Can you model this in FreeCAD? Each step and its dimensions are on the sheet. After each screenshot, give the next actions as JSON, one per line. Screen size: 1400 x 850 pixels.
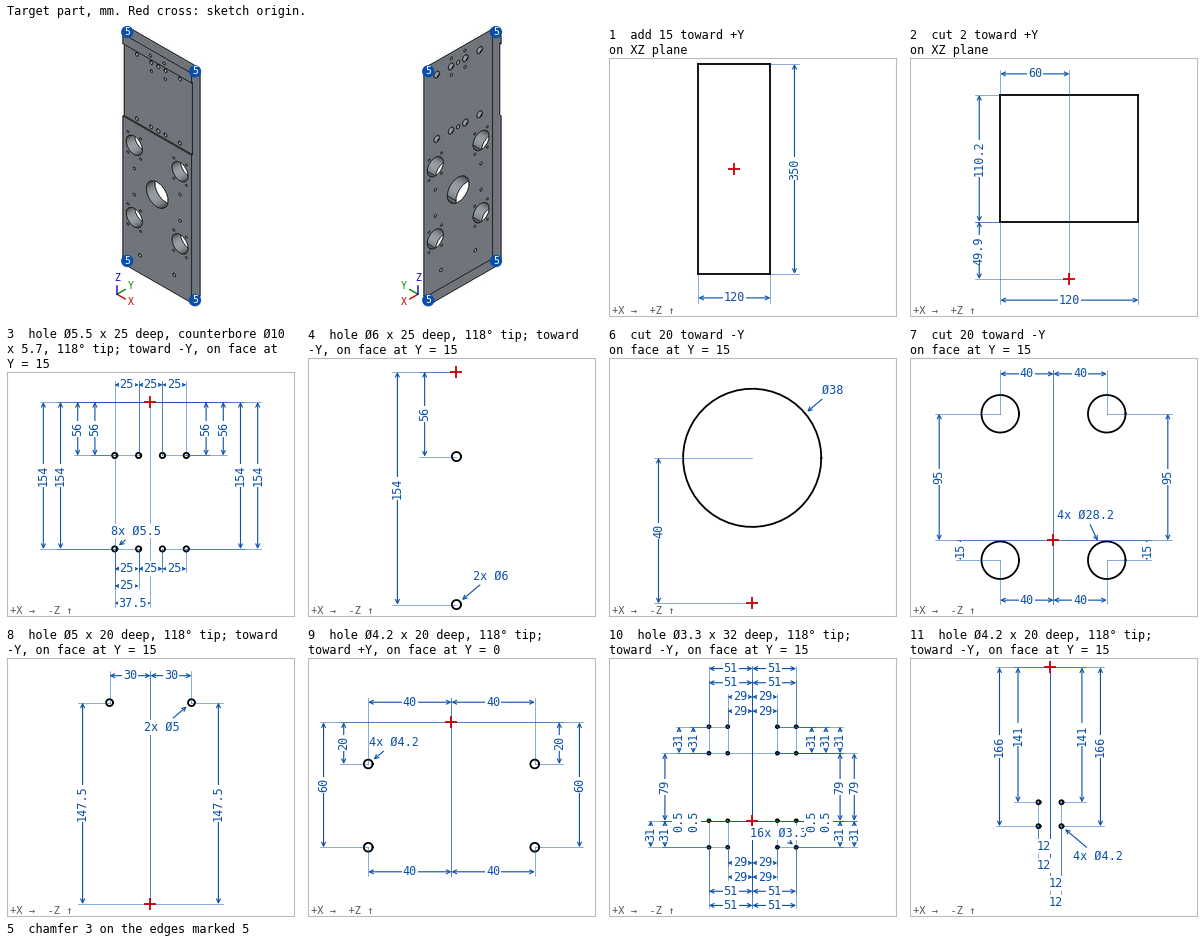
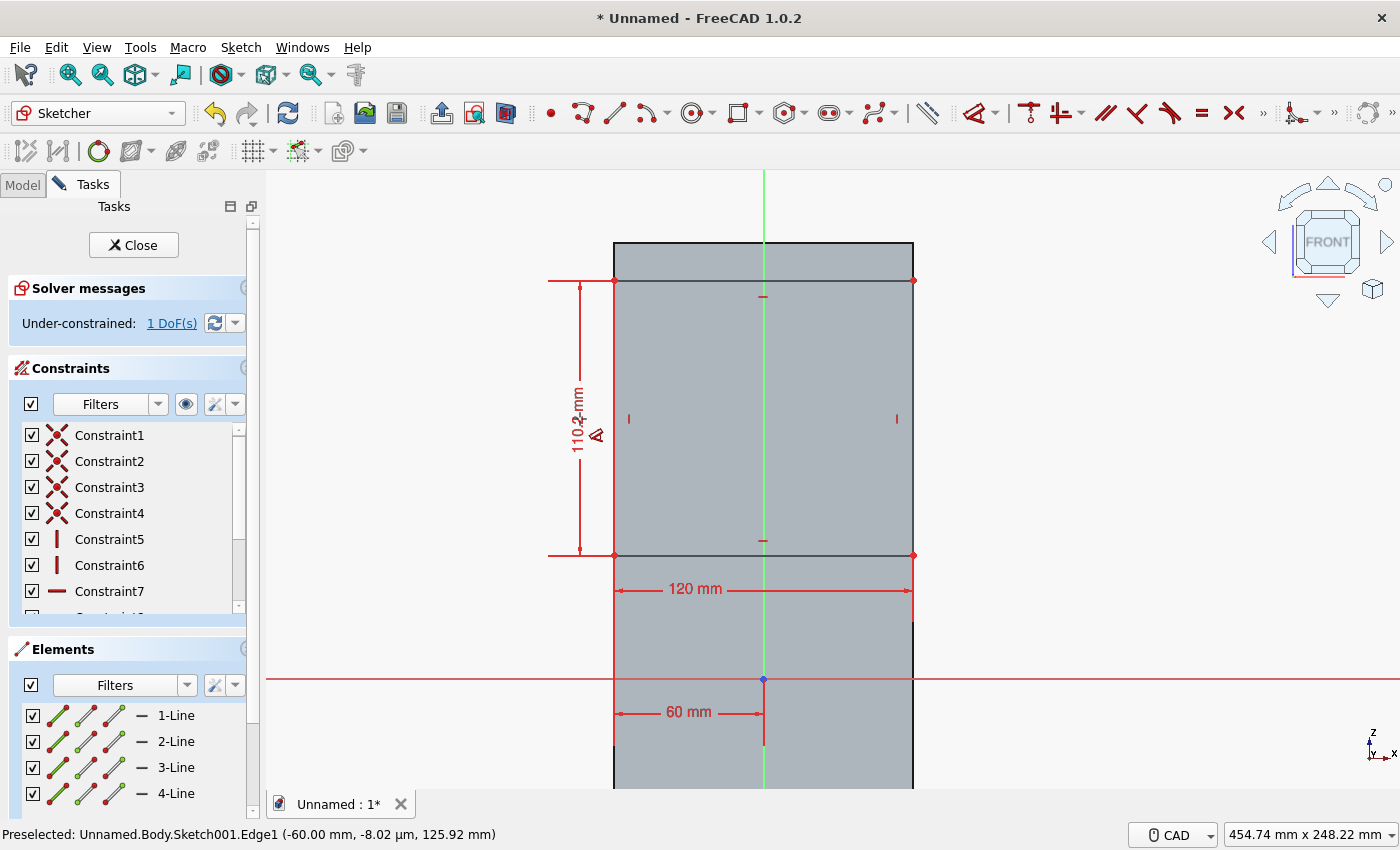
{"action": "left_click", "coordinate": [614, 556]}
{"action": "left_click", "coordinate": [580, 617]}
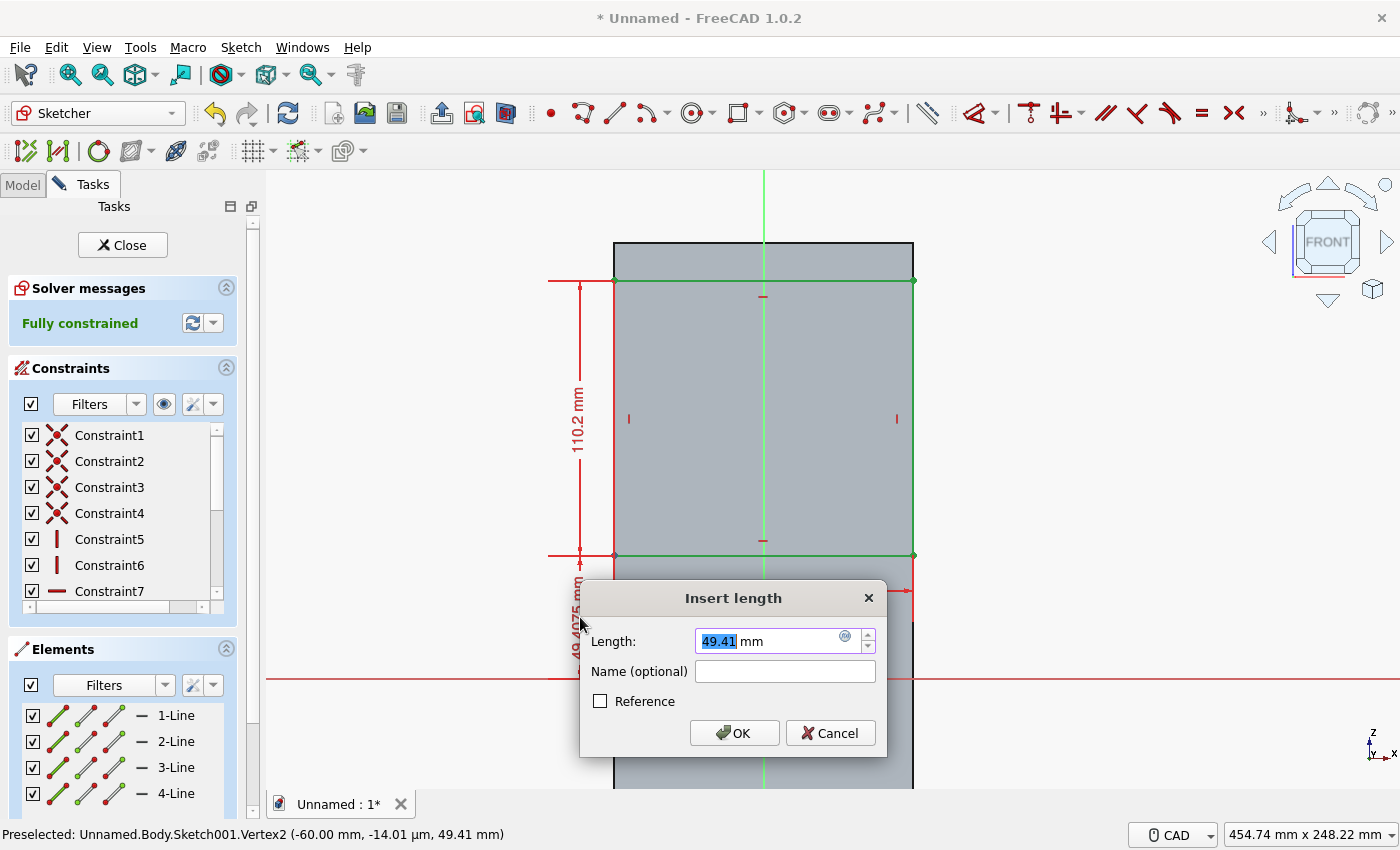
{"action": "type", "text": "49.9"}
{"action": "key", "text": "Return"}
{"action": "key", "text": "Escape"}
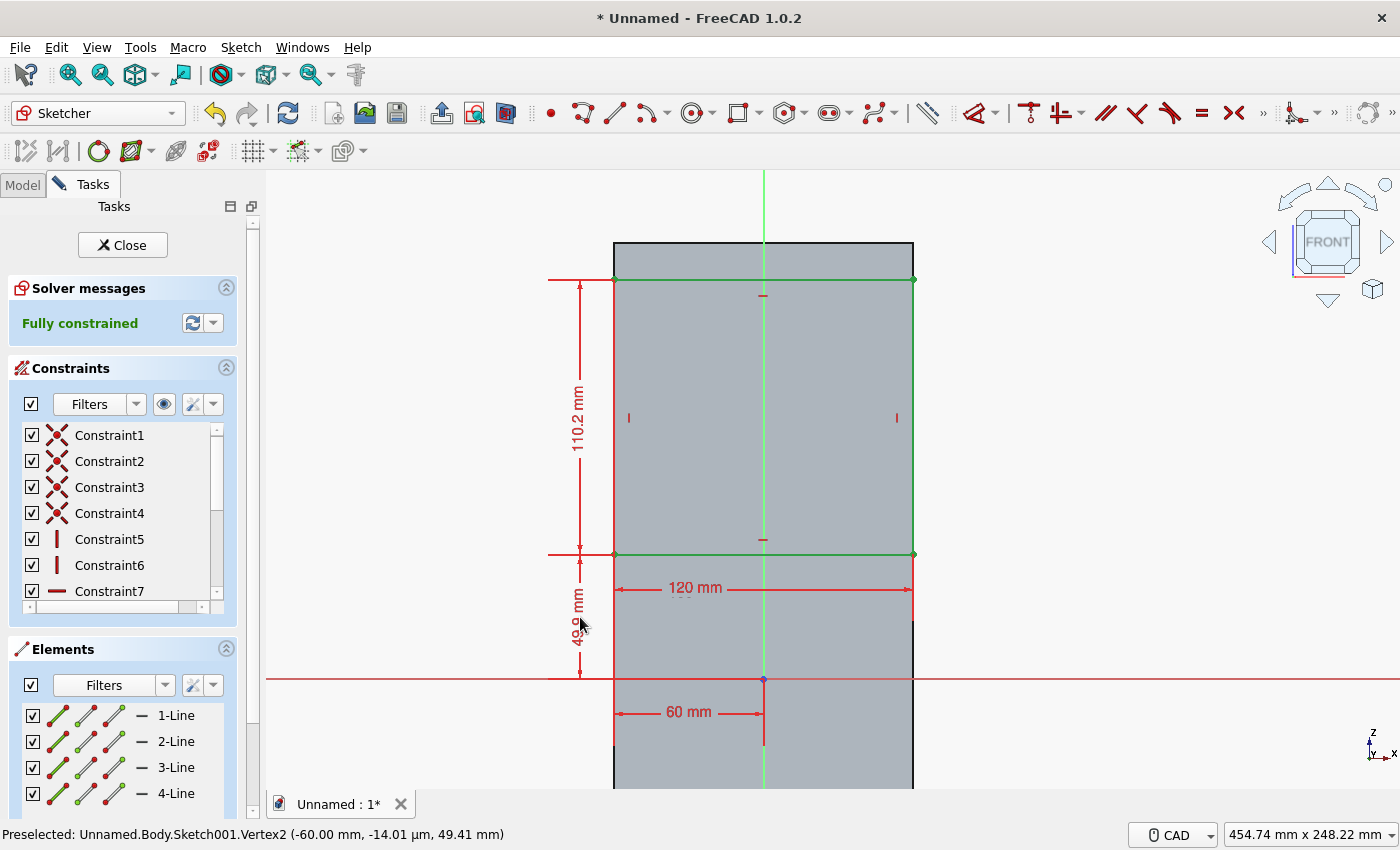
{"action": "left_click", "coordinate": [123, 245]}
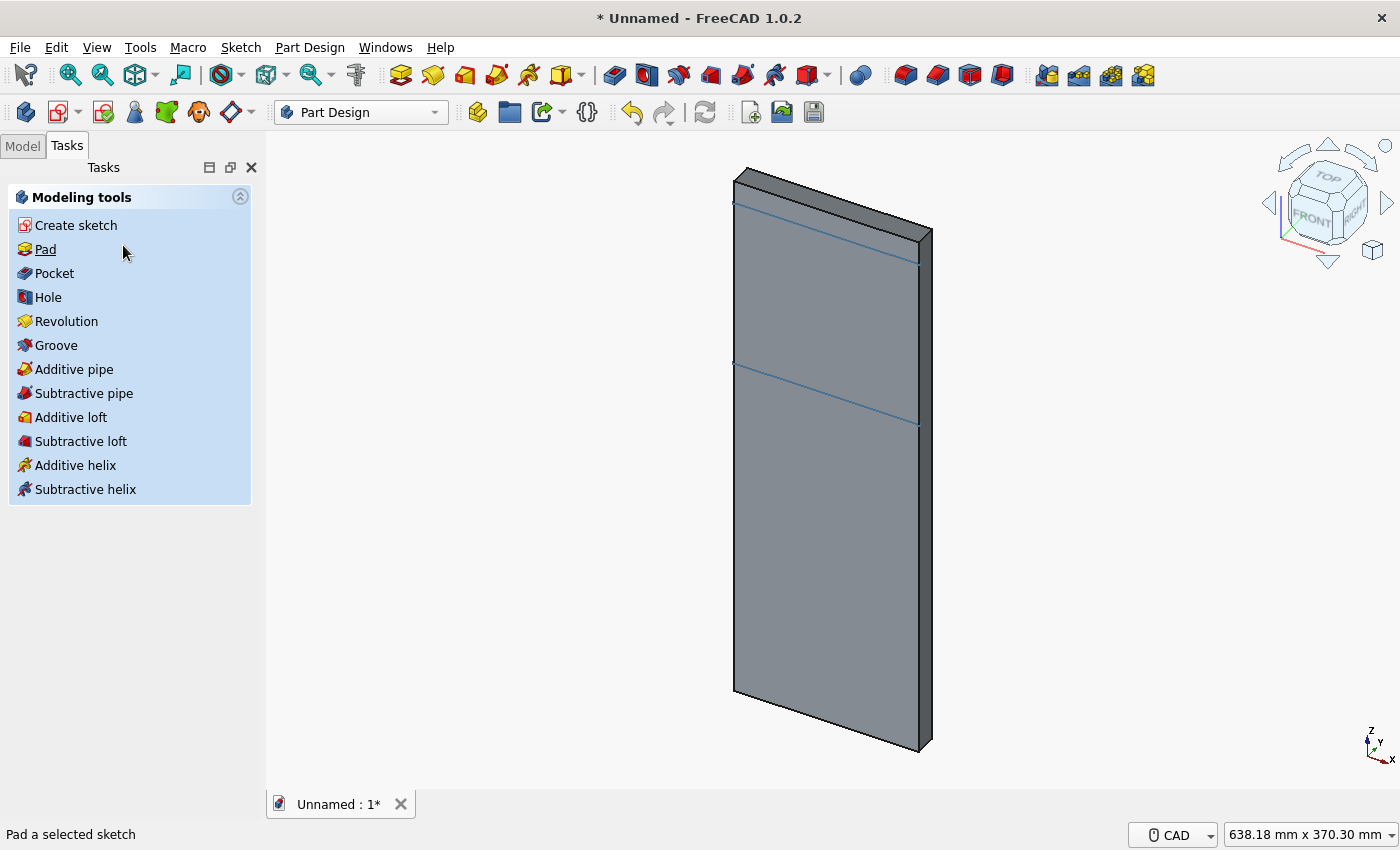
{"action": "left_click", "coordinate": [616, 76]}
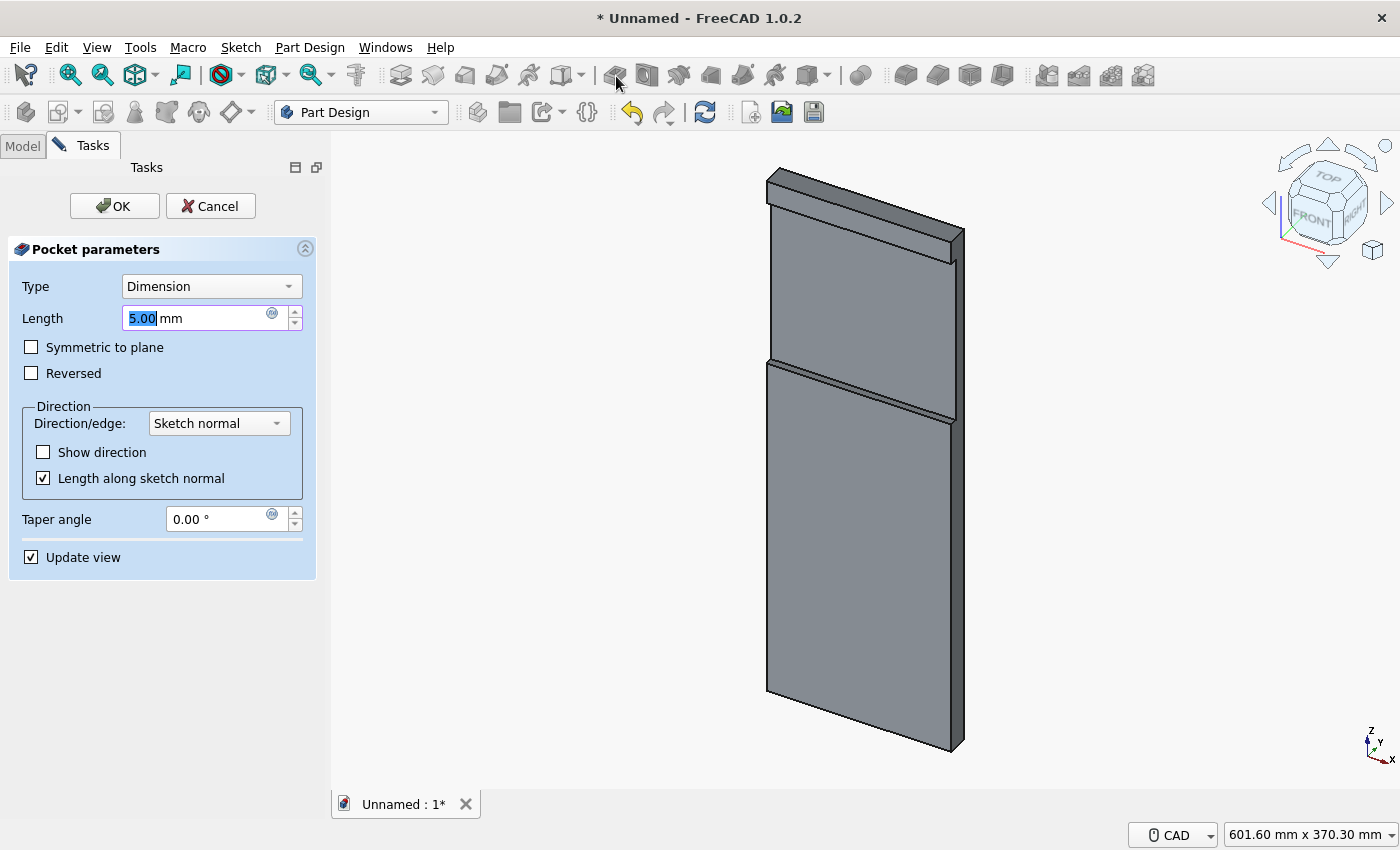
{"action": "type", "text": "2"}
{"action": "key", "text": "Tab"}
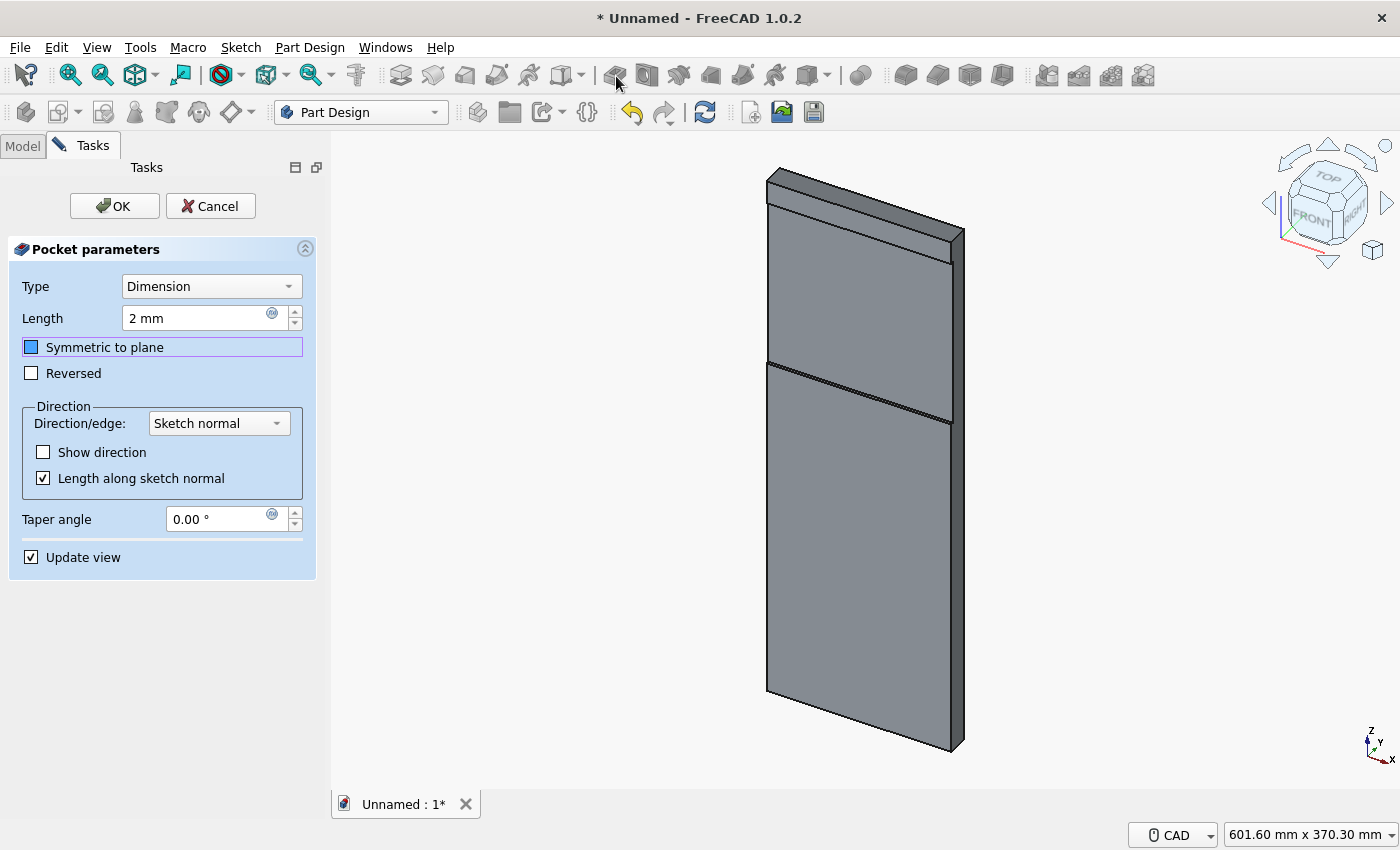
{"action": "left_click", "coordinate": [115, 206]}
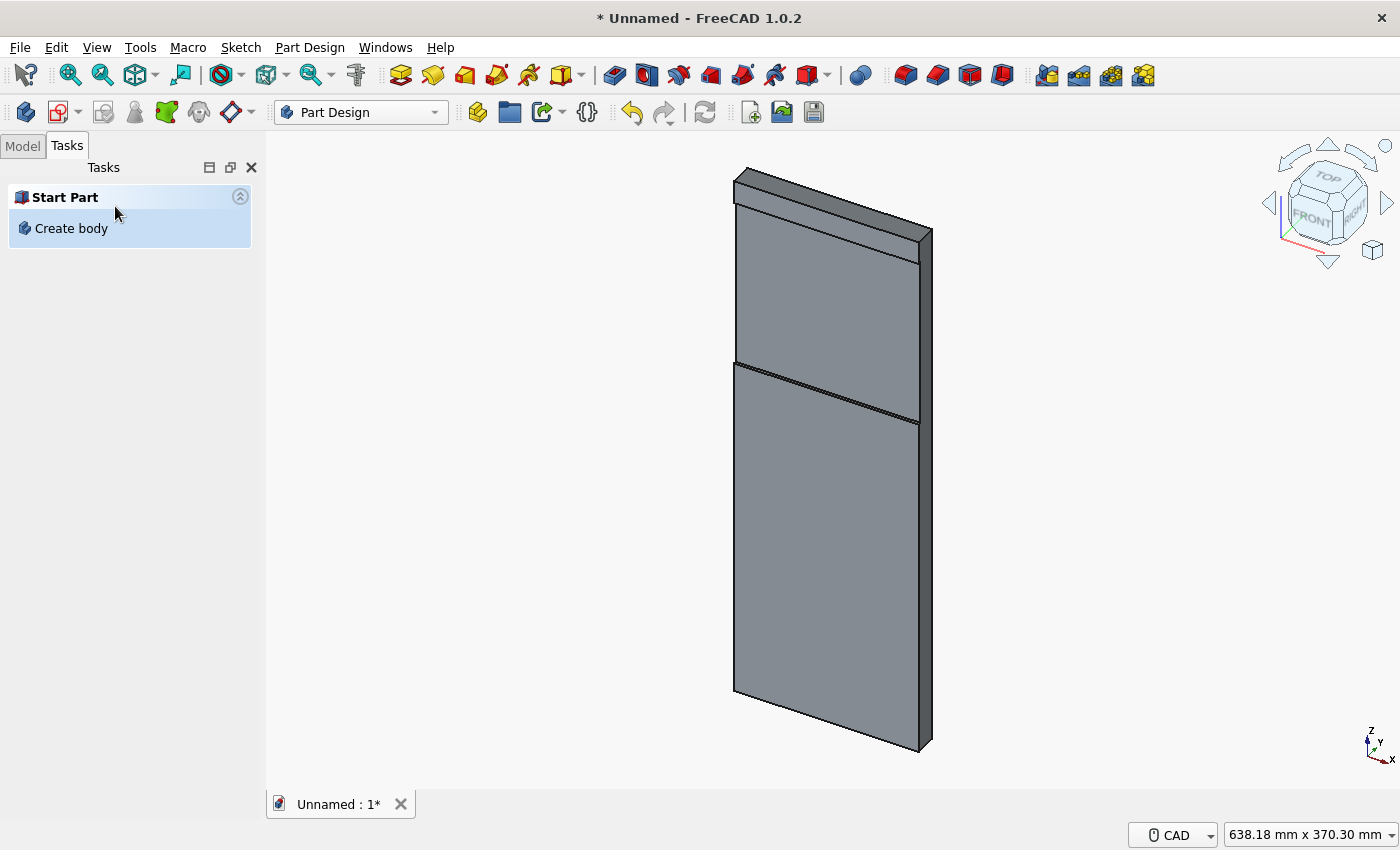
{"action": "key", "text": "4"}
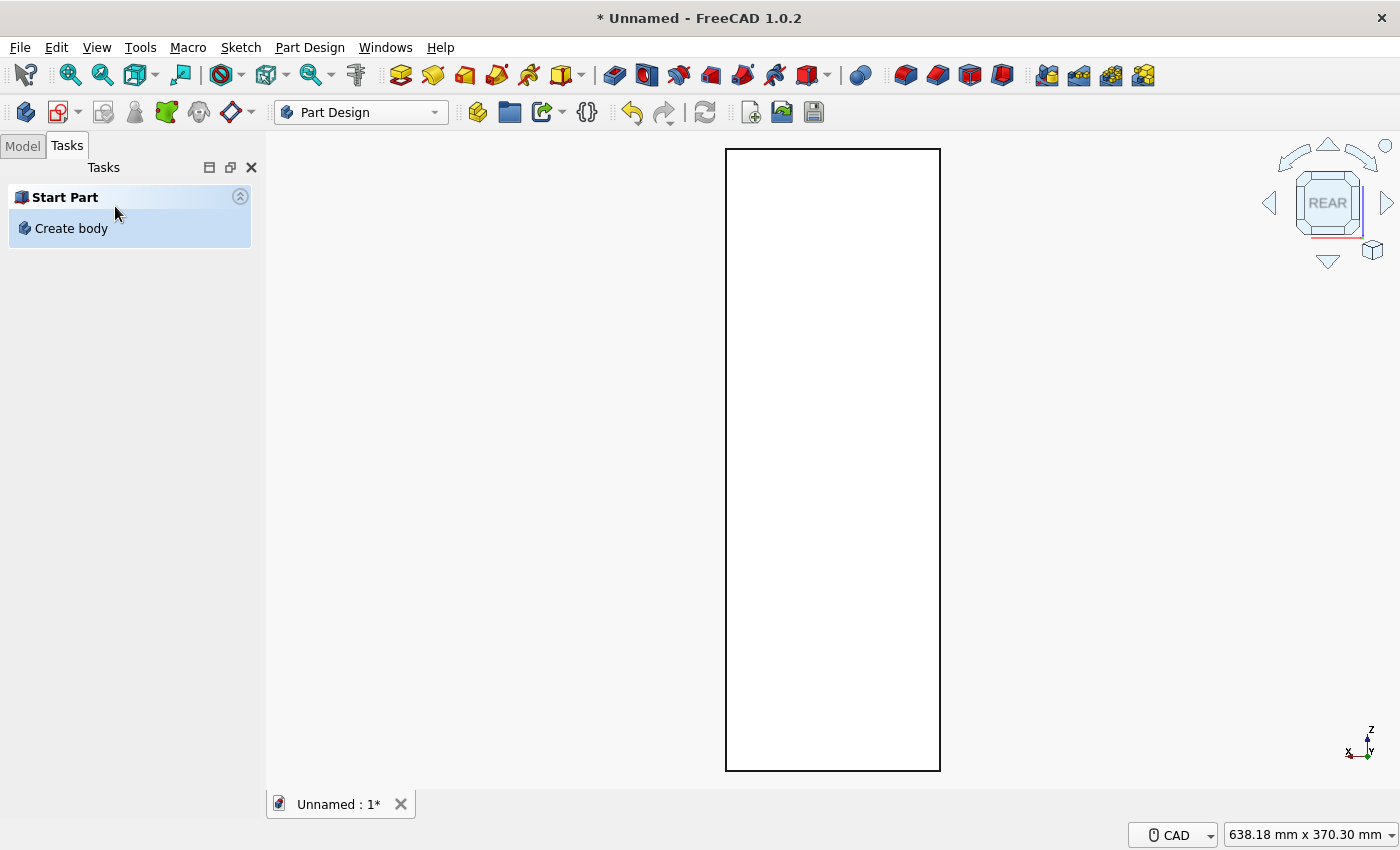
{"action": "left_click", "coordinate": [833, 281]}